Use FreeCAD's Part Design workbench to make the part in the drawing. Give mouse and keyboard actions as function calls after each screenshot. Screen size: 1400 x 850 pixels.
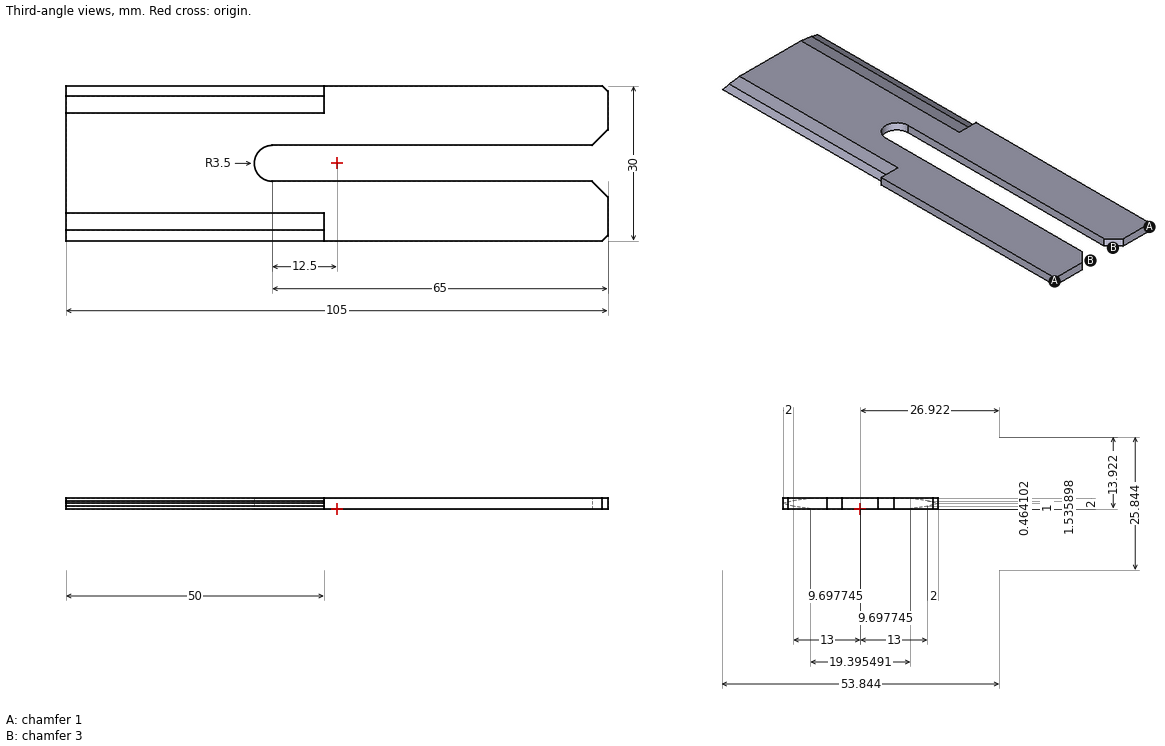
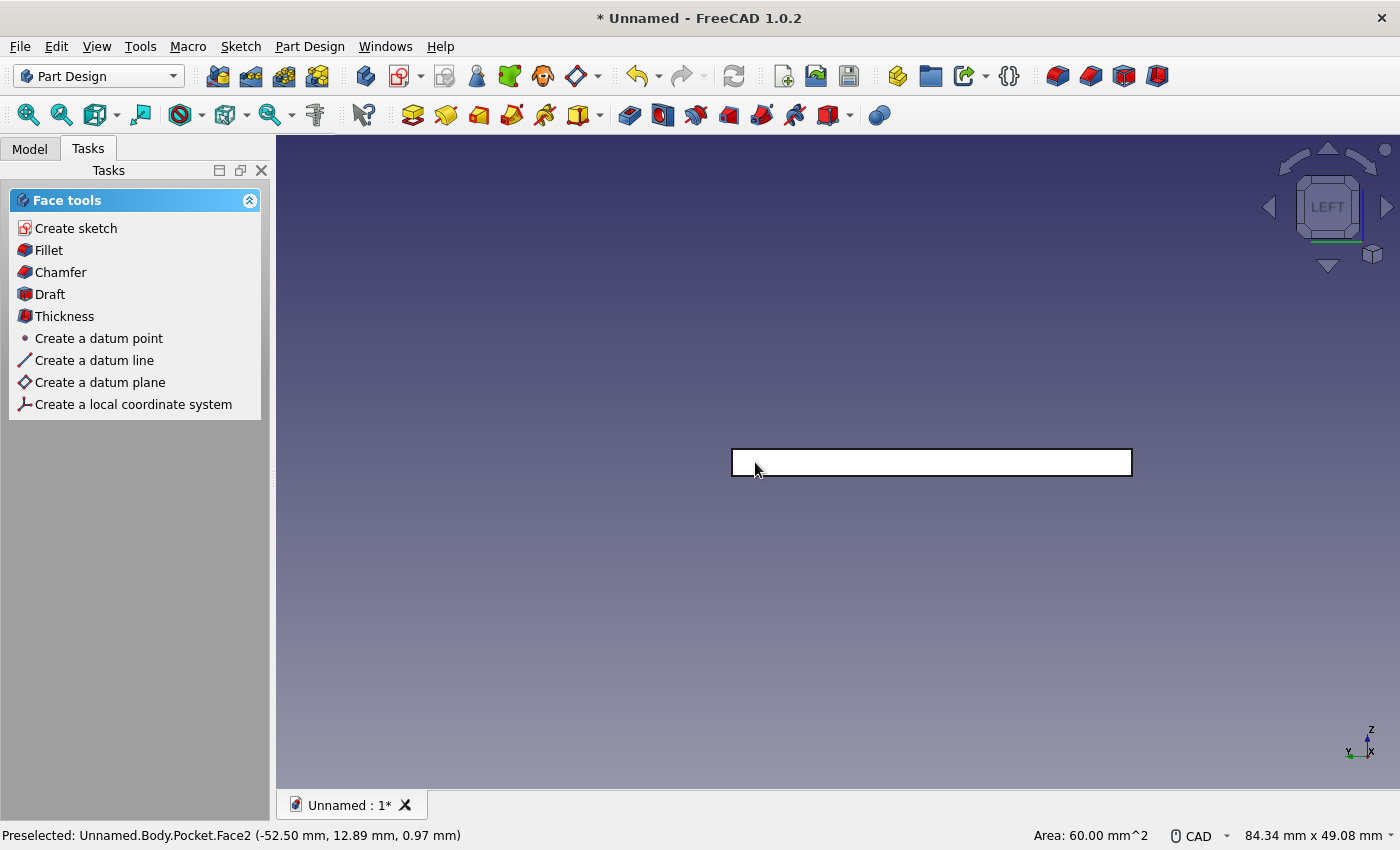
click(398, 76)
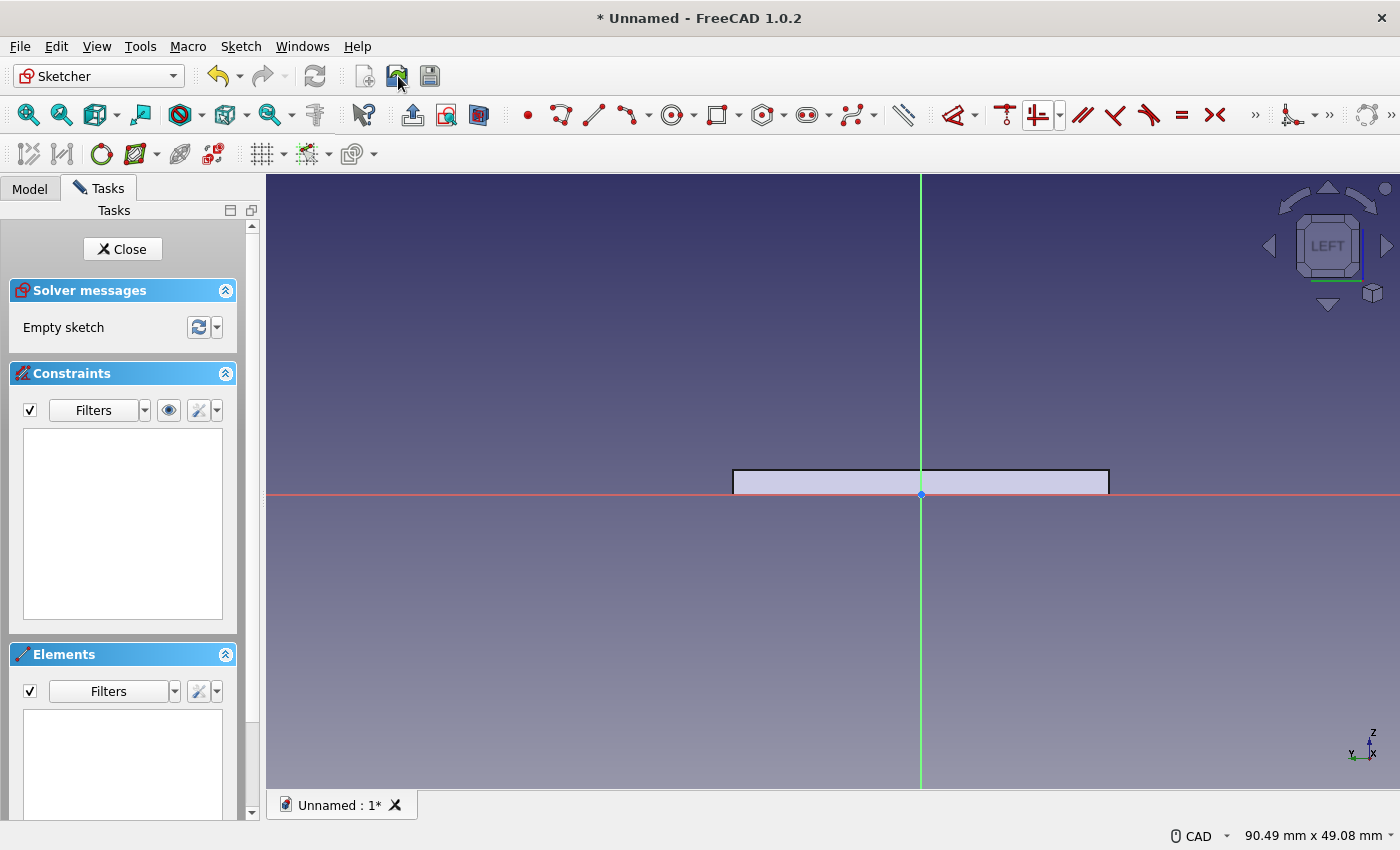
scroll(294, 479, down, 1)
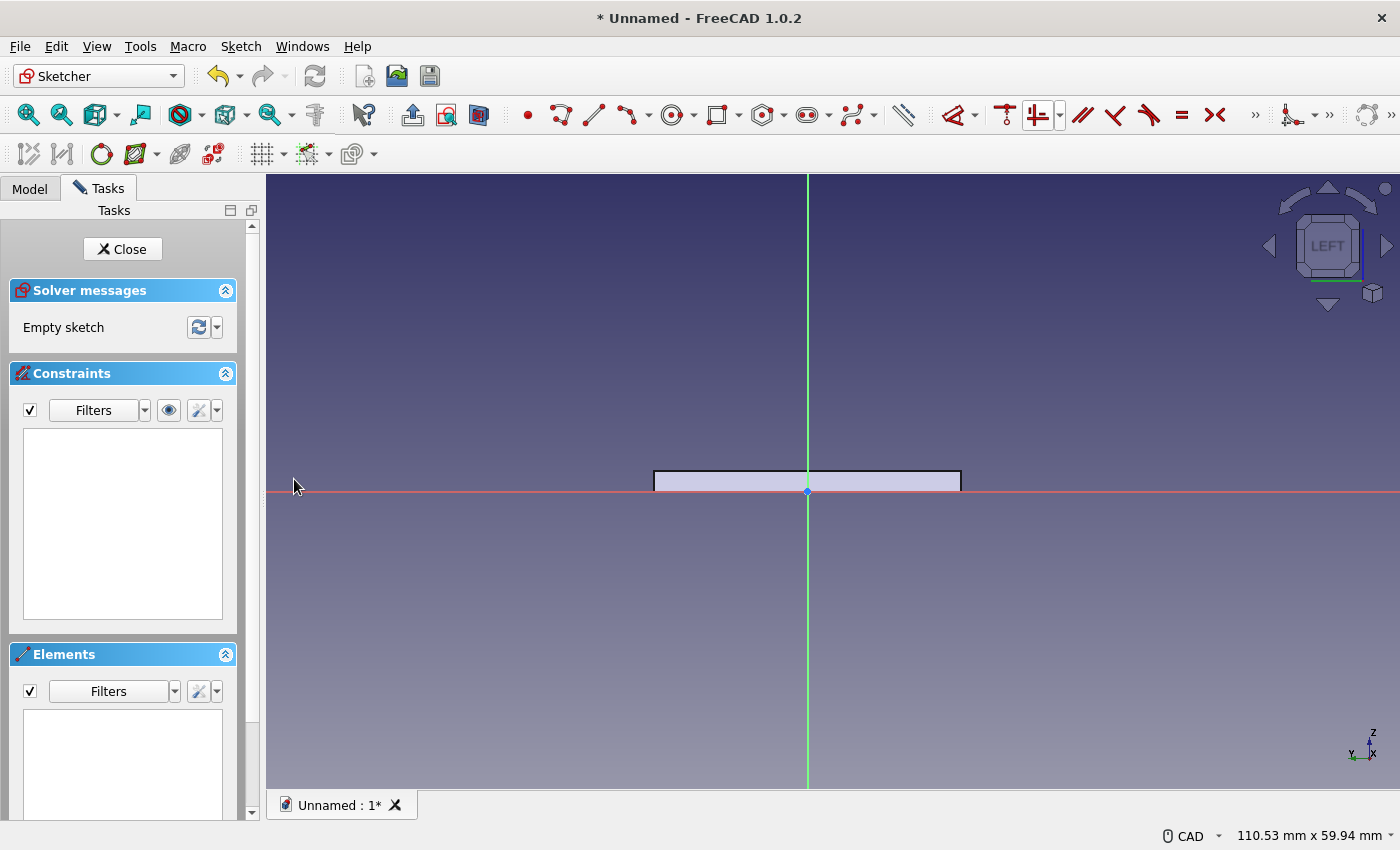
click(716, 116)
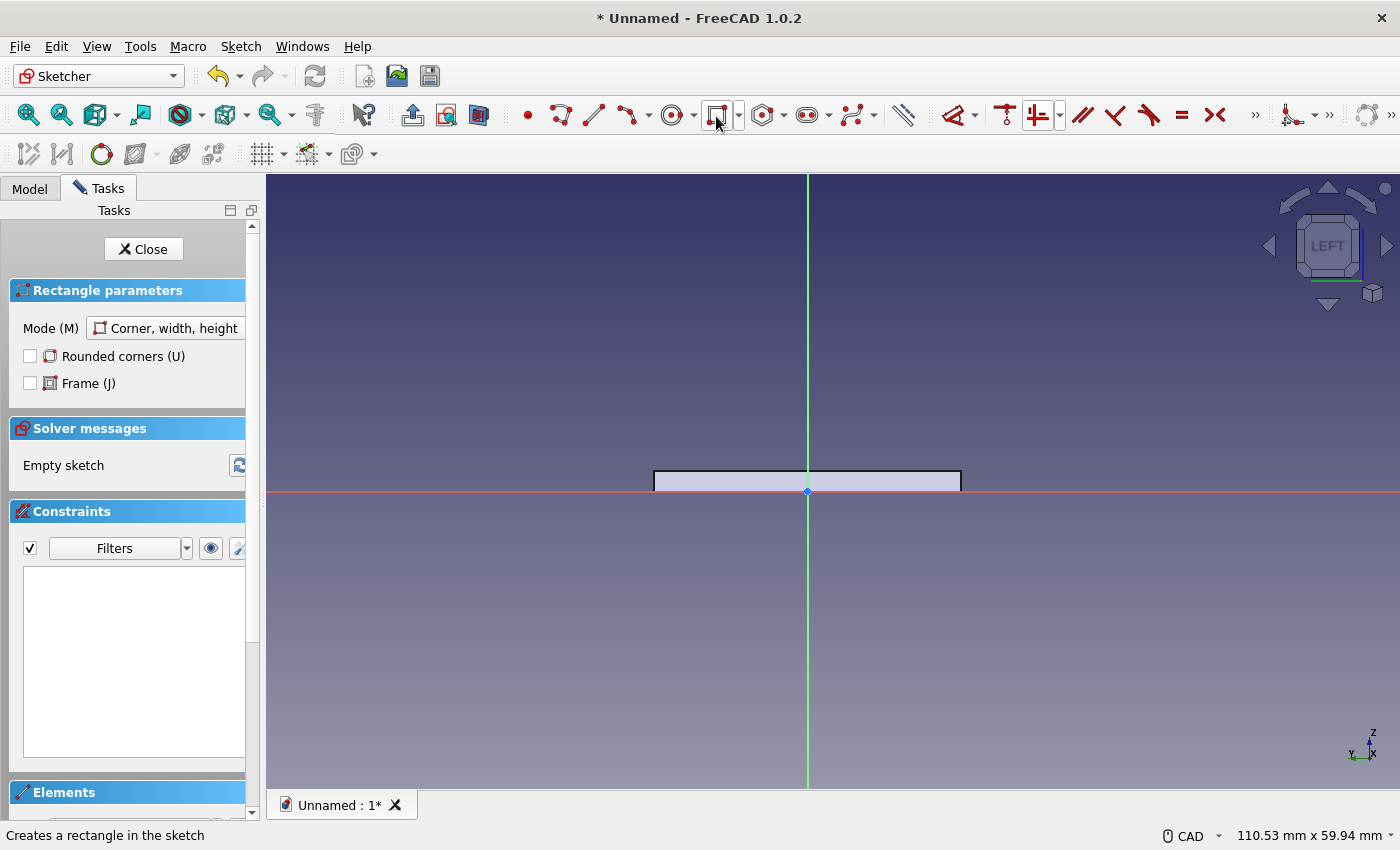
click(531, 349)
click(1084, 614)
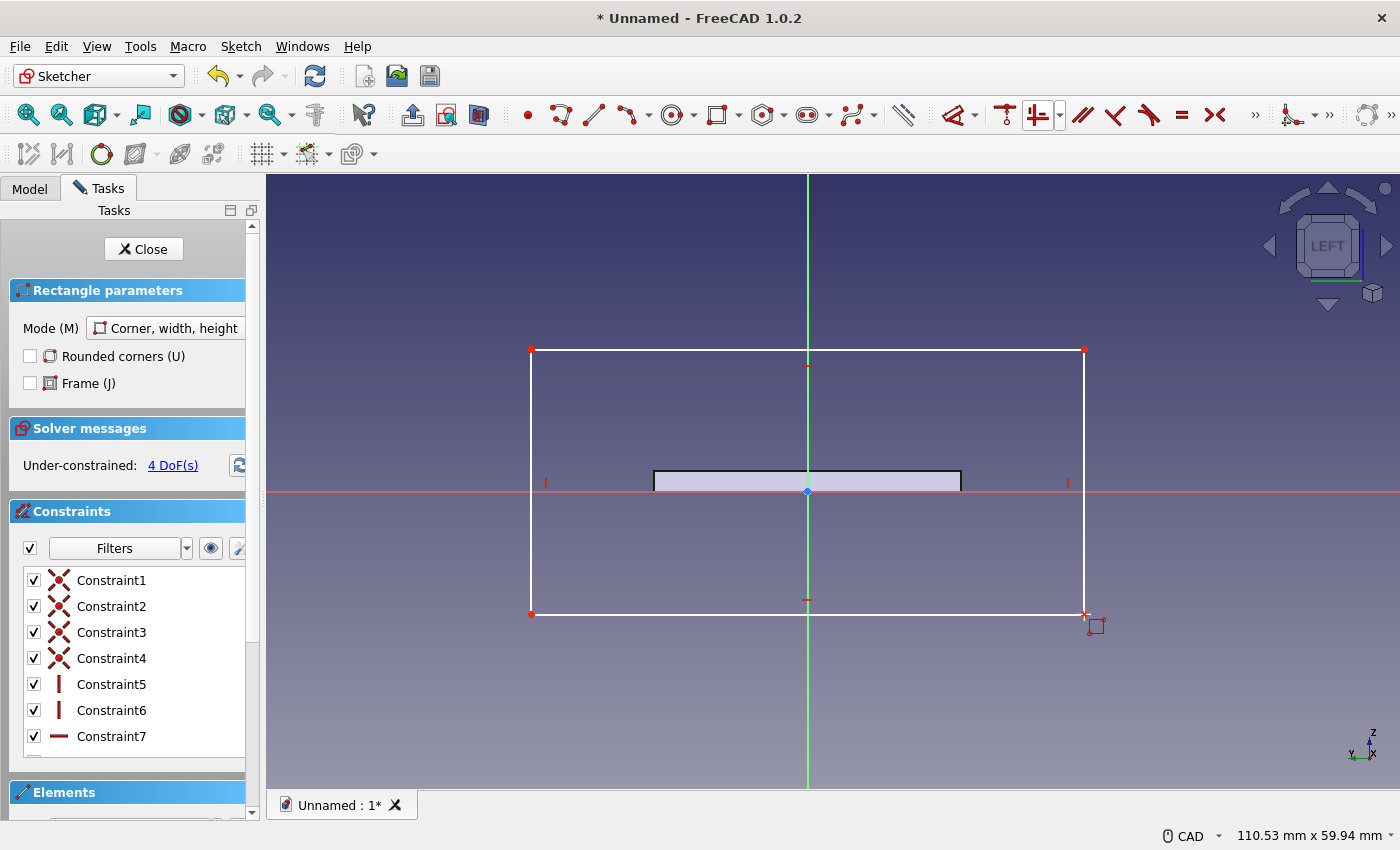
click(561, 116)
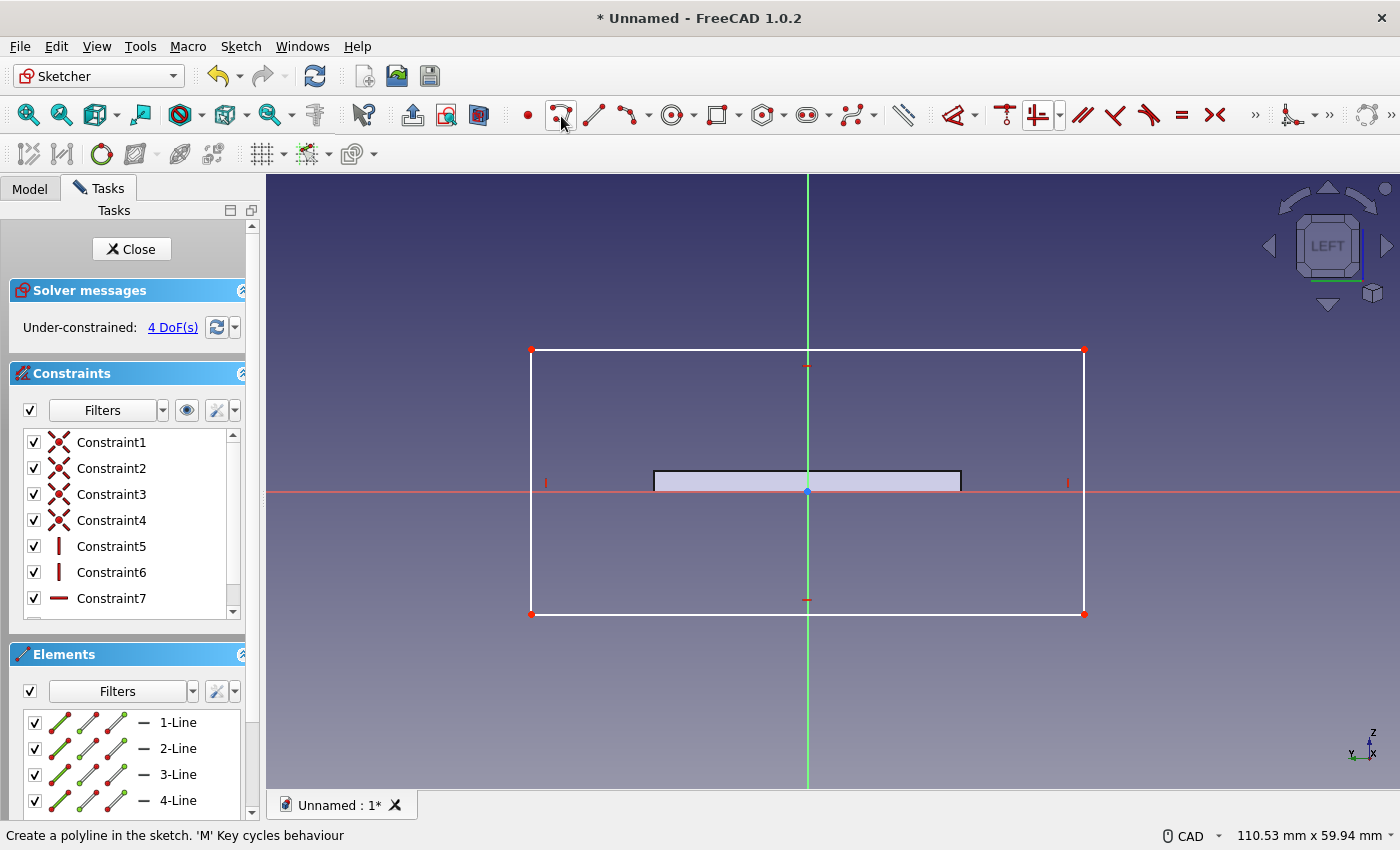
click(907, 492)
click(708, 483)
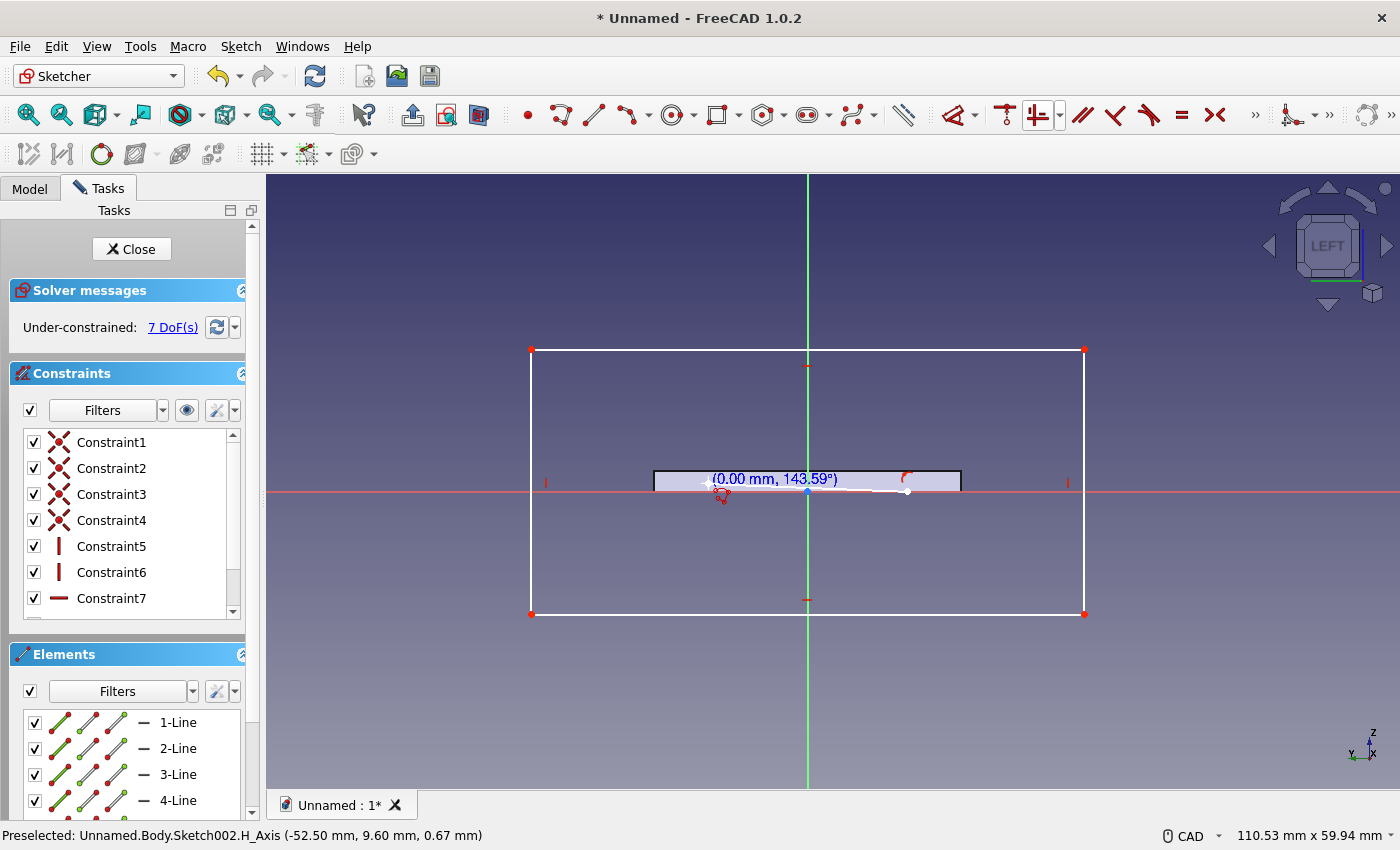
scroll(674, 487, up, 7)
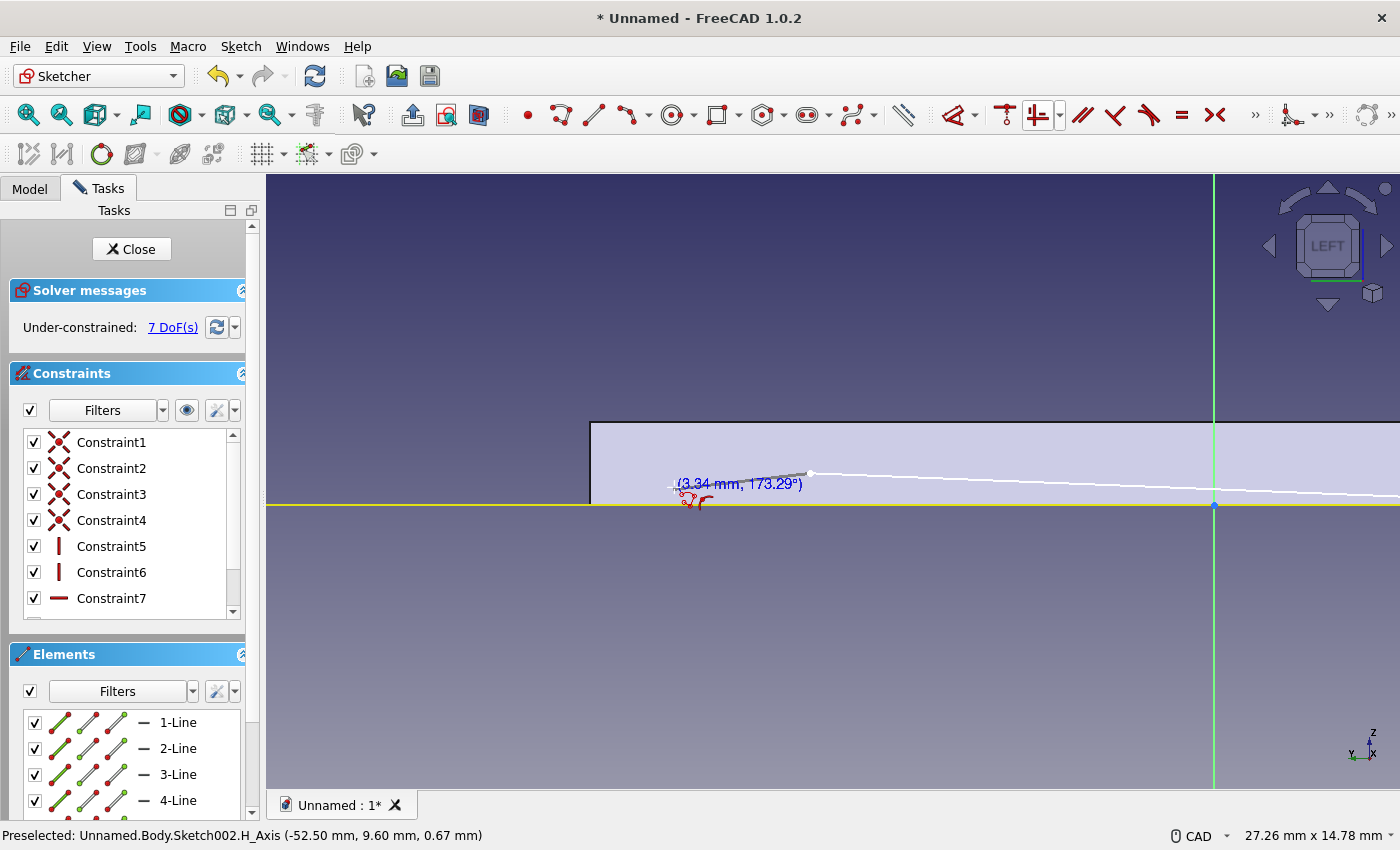
click(674, 486)
click(590, 464)
click(674, 441)